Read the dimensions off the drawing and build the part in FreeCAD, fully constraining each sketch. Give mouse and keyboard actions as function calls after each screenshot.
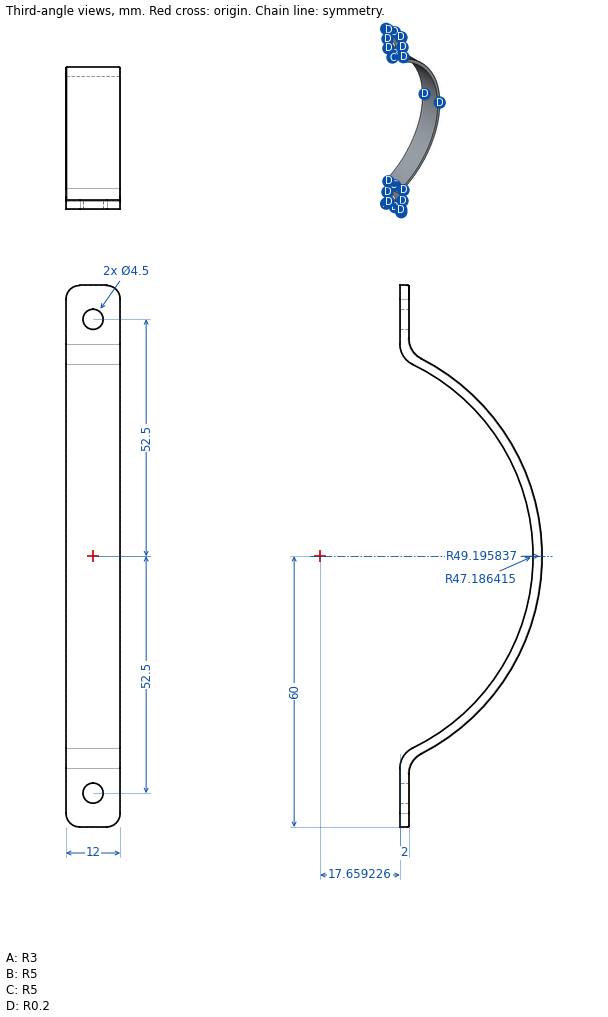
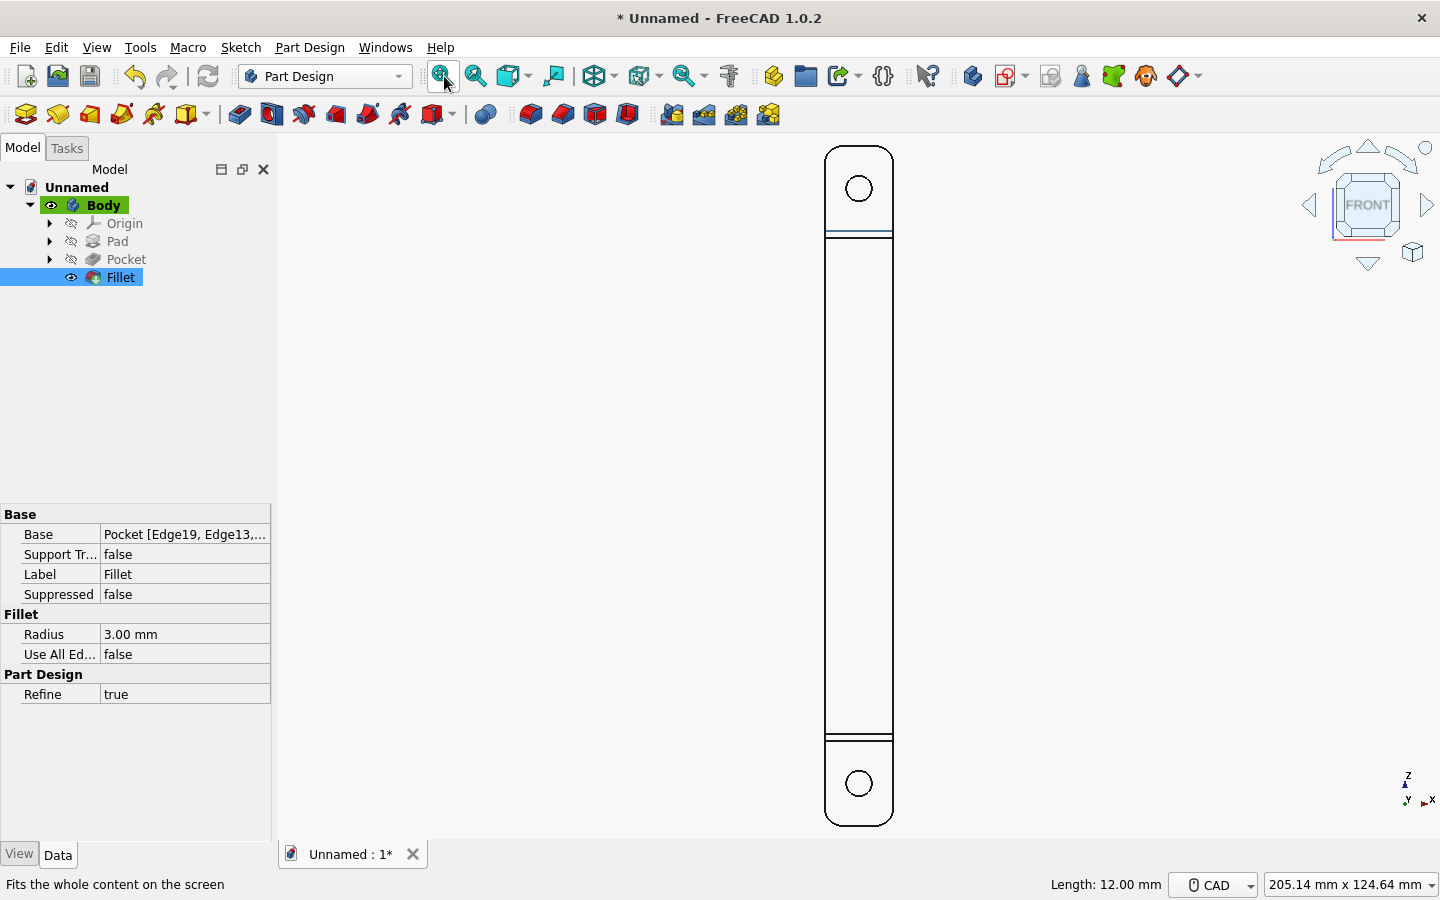
click(859, 740, ctrl)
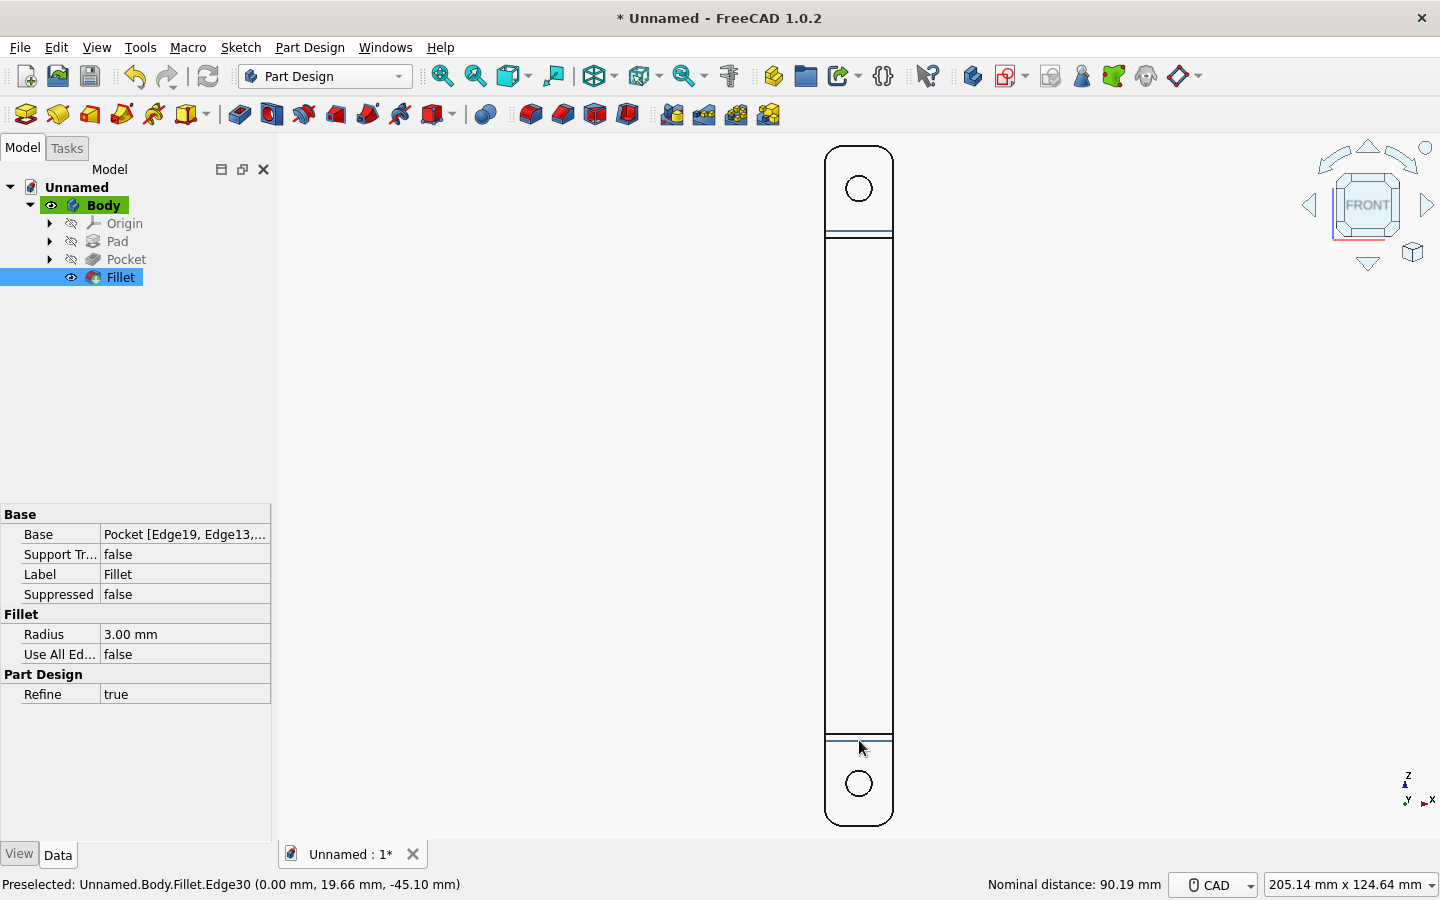
key(v)
key(1)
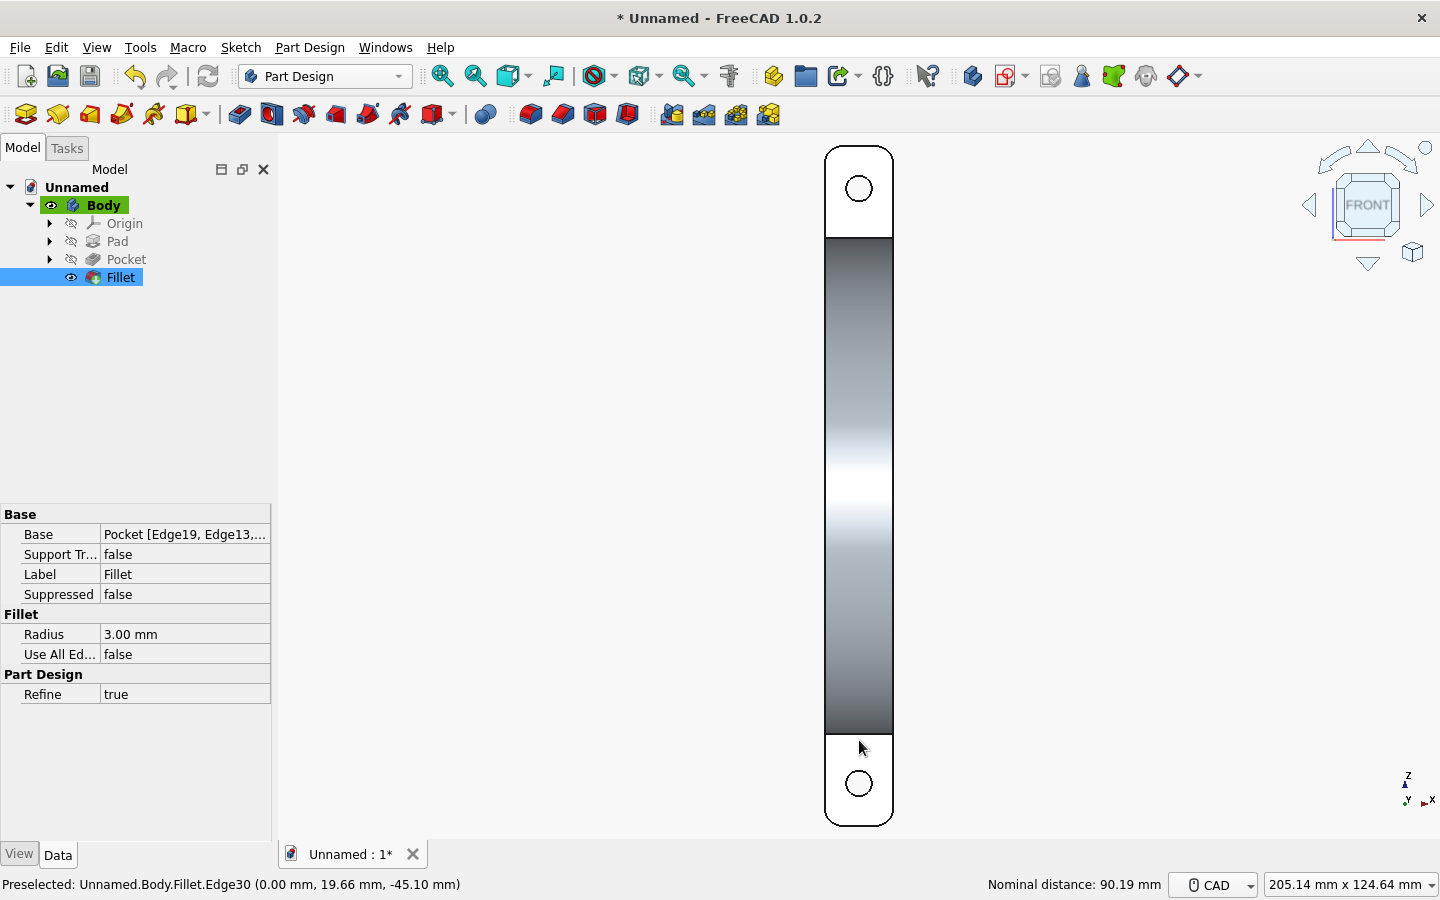
click(532, 114)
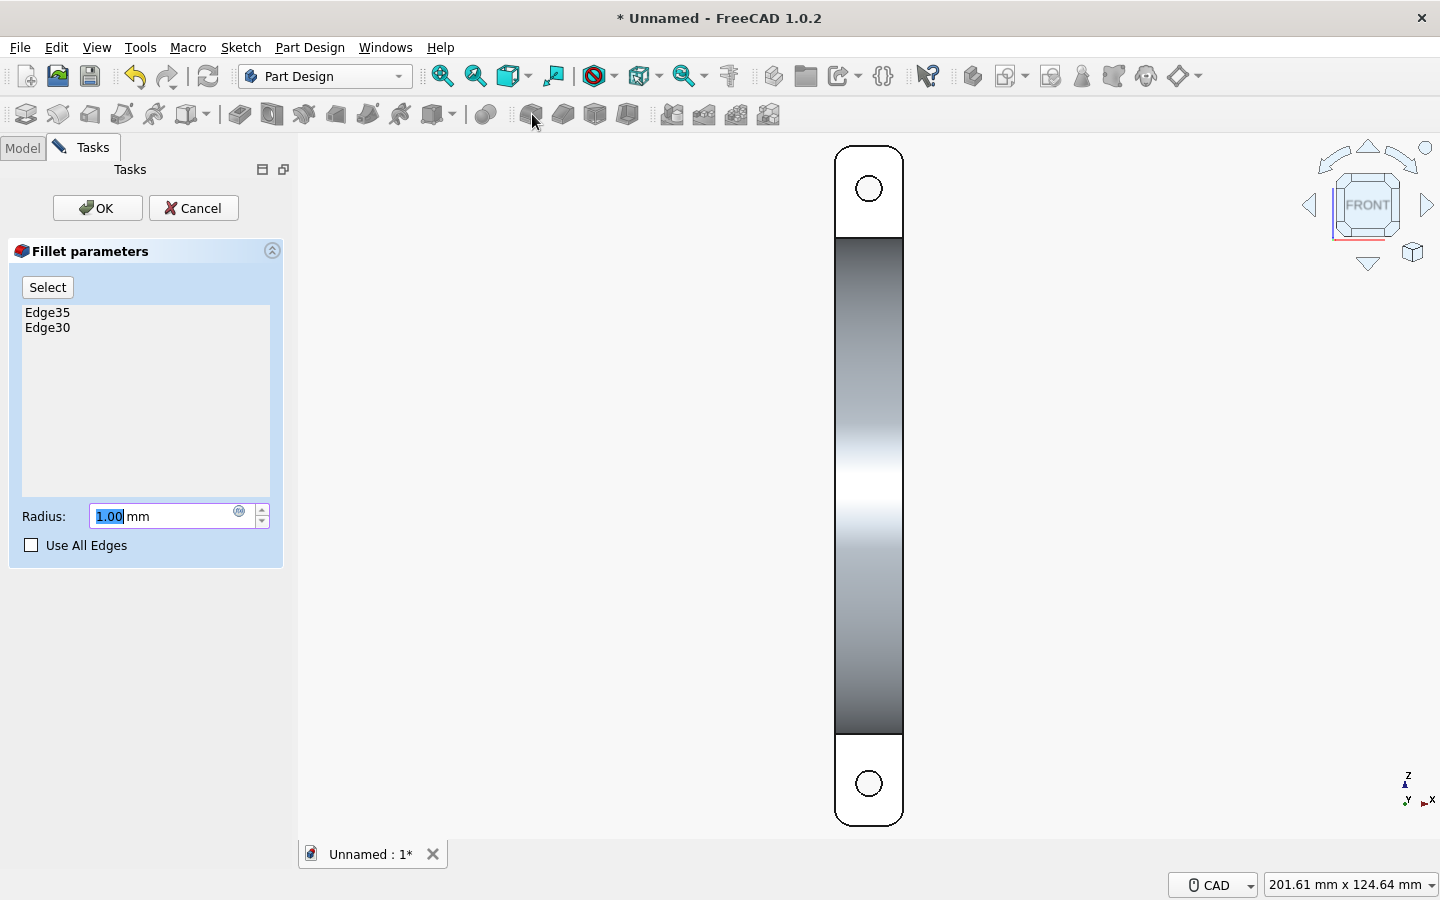
text(5)
key(Tab)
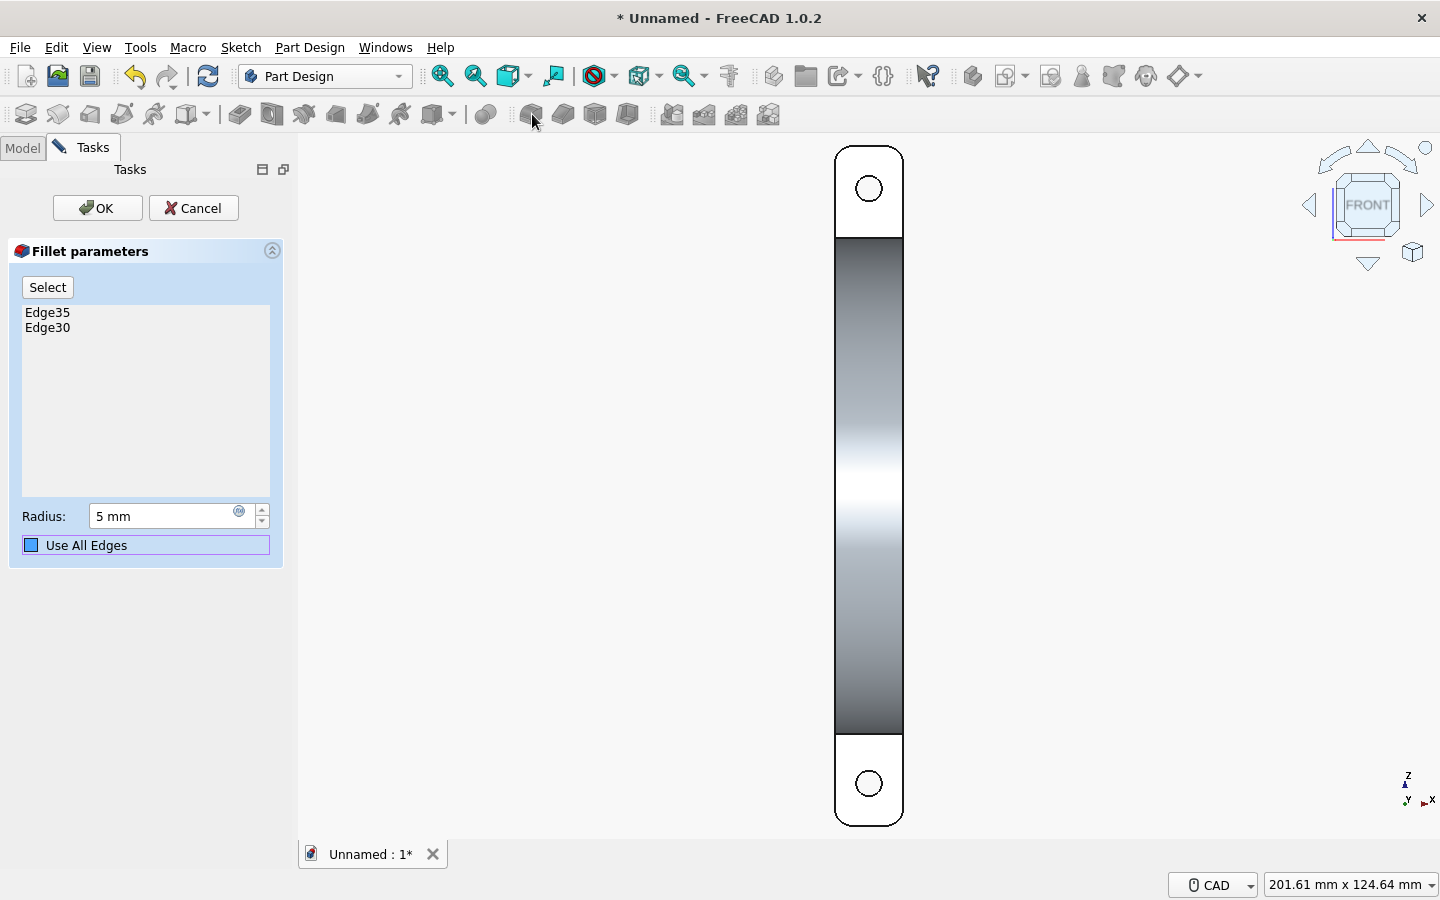
click(98, 208)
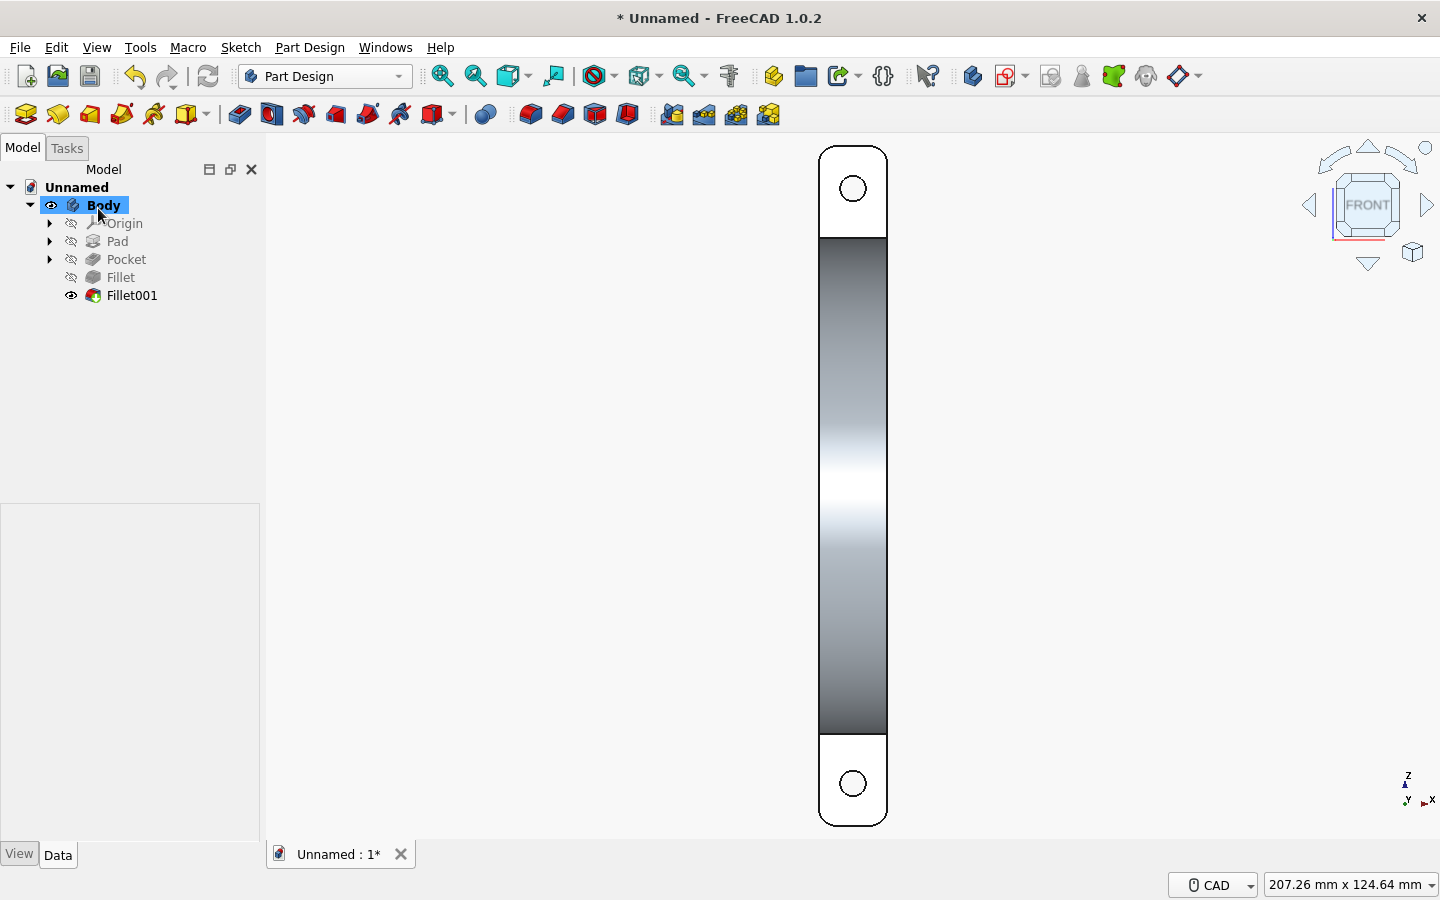
click(853, 237)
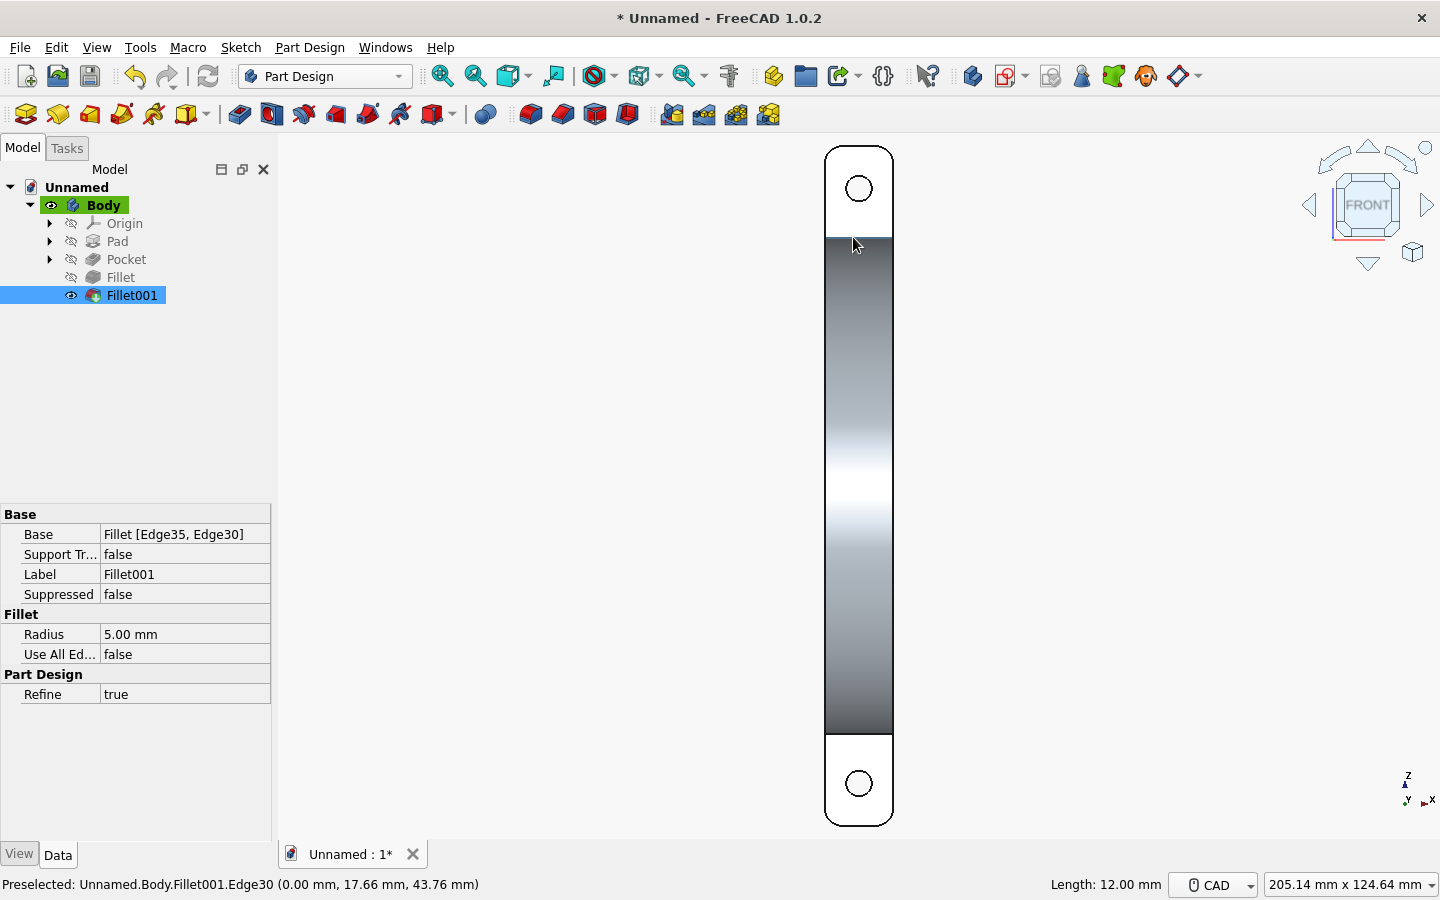
click(859, 733, ctrl)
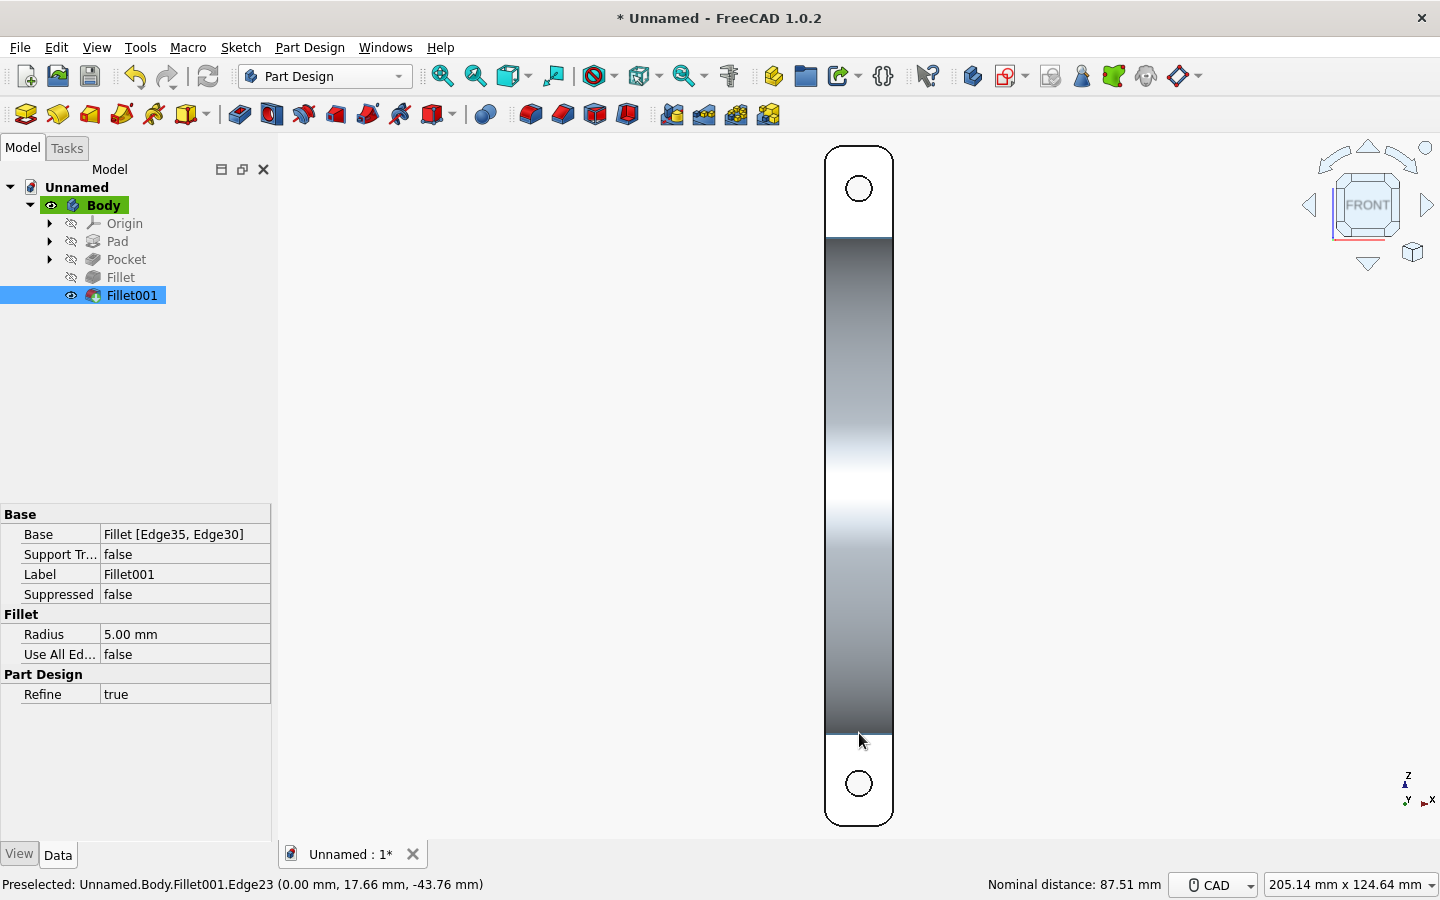
click(532, 114)